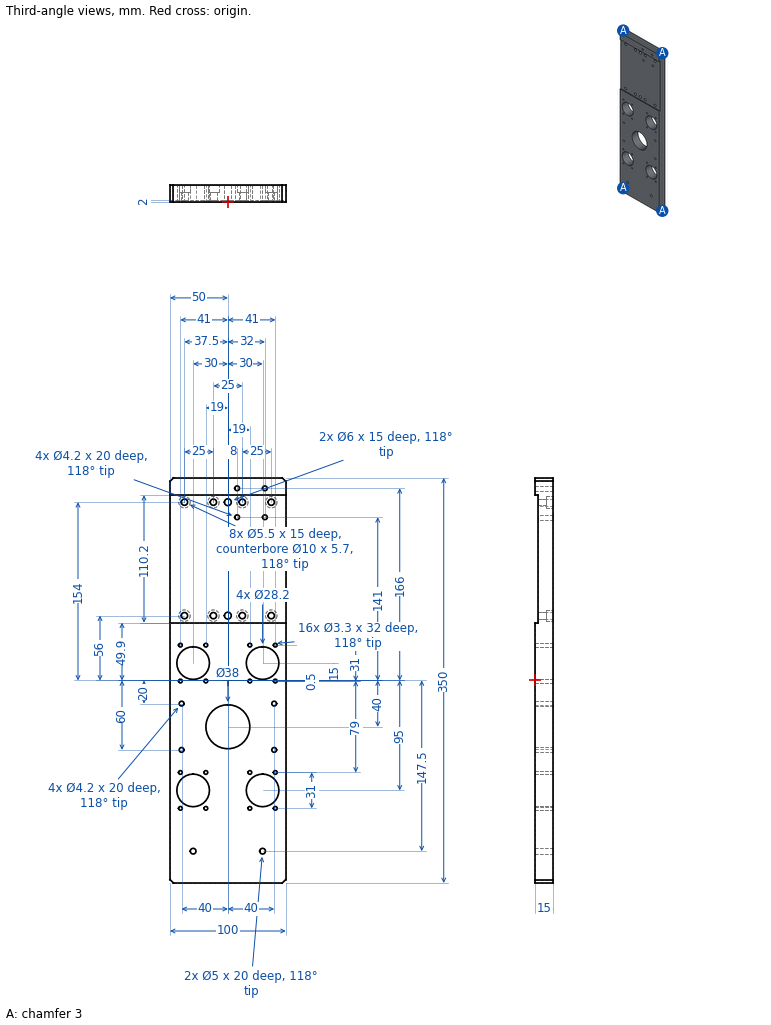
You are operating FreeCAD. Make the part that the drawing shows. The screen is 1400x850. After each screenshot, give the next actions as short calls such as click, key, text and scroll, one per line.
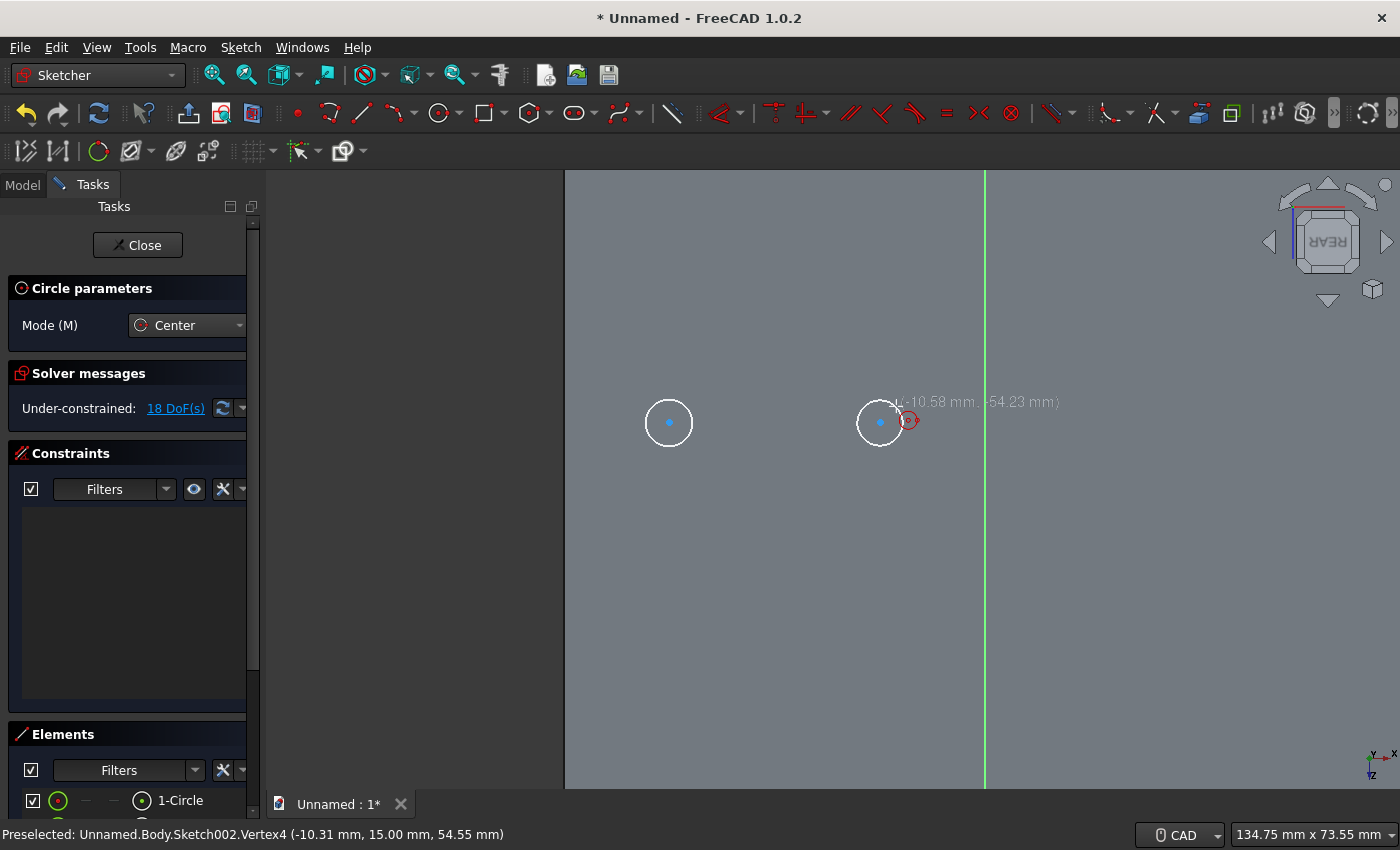
click(1090, 422)
click(1107, 406)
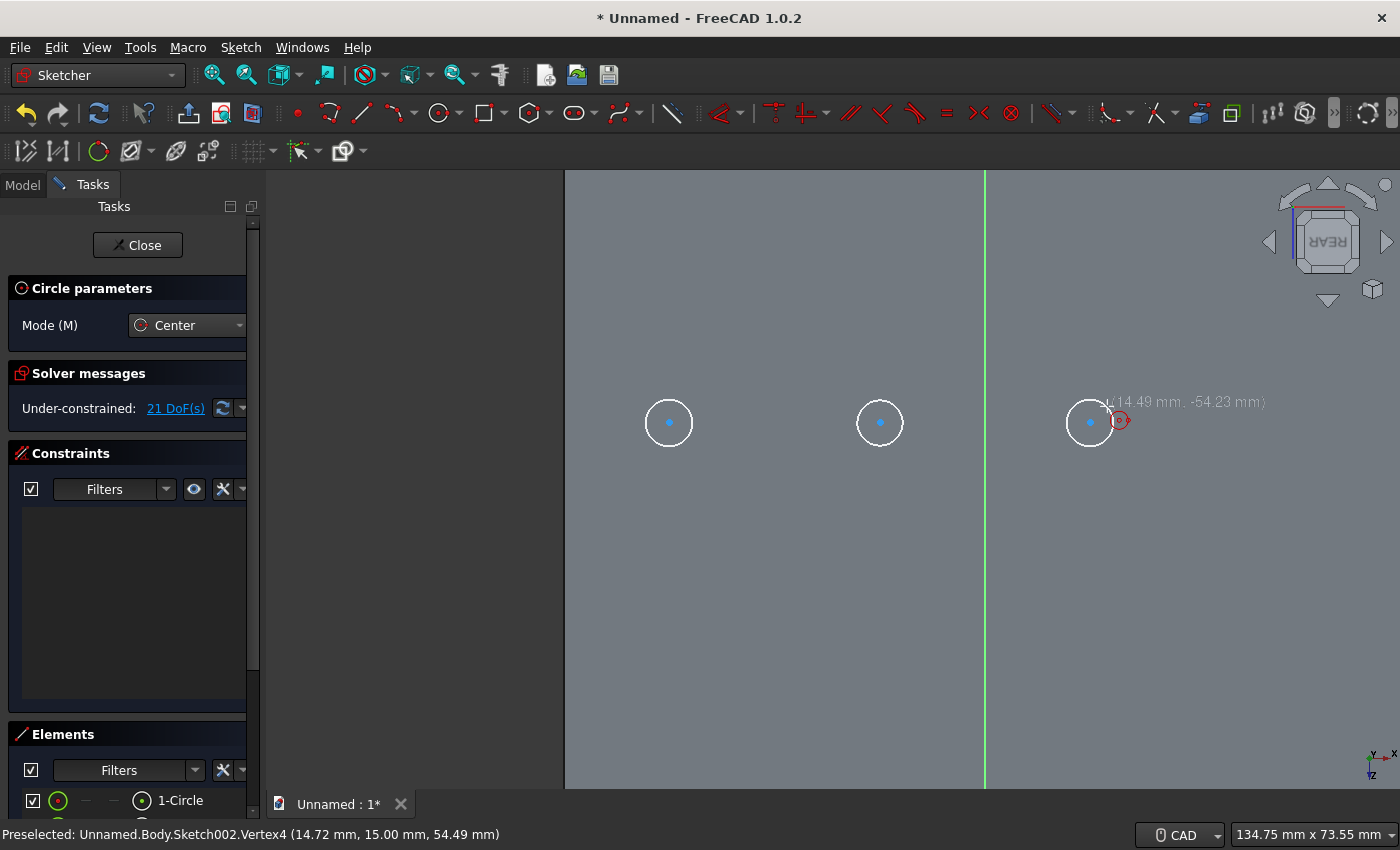
scroll(669, 423, down, 6)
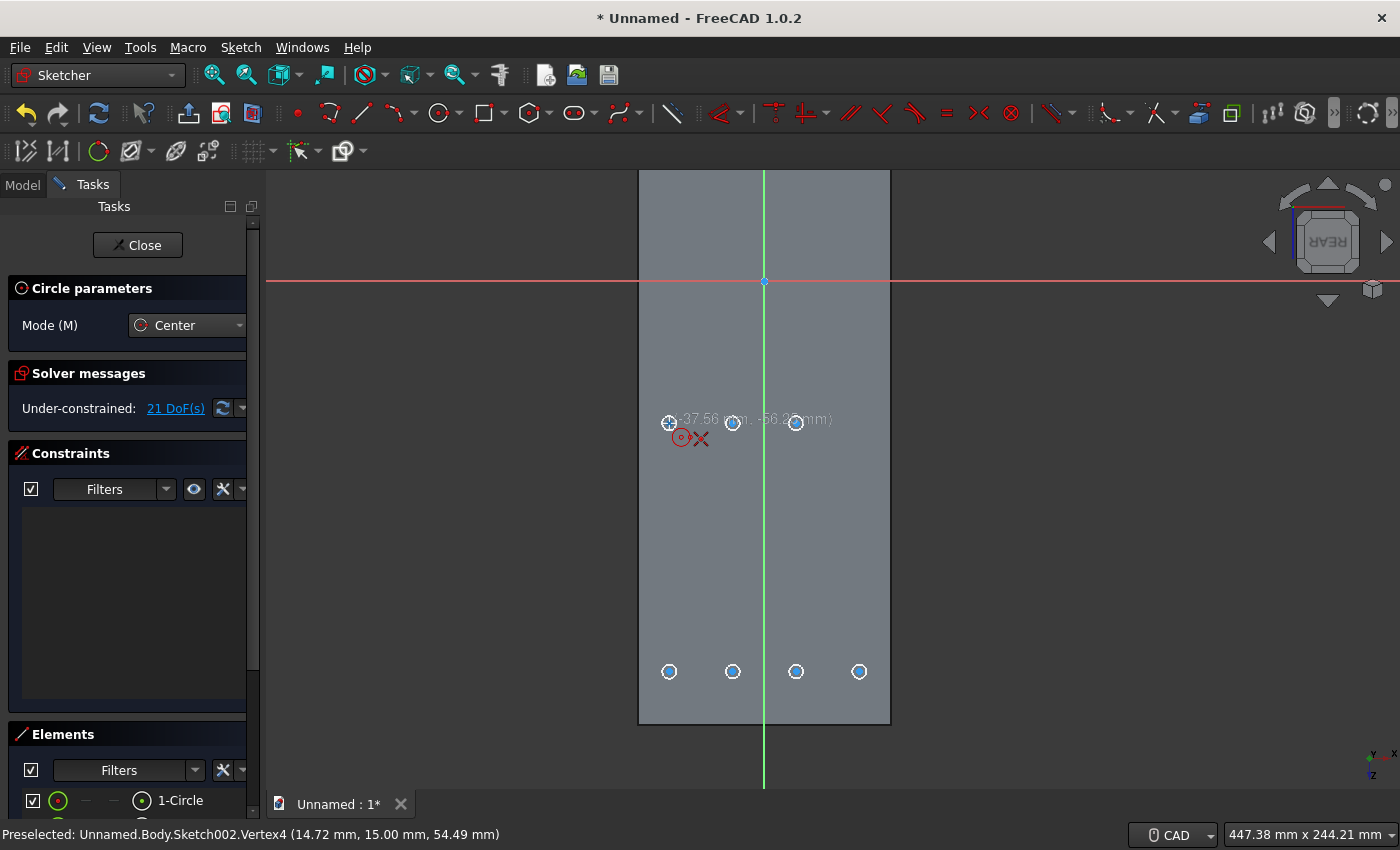
scroll(859, 423, up, 6)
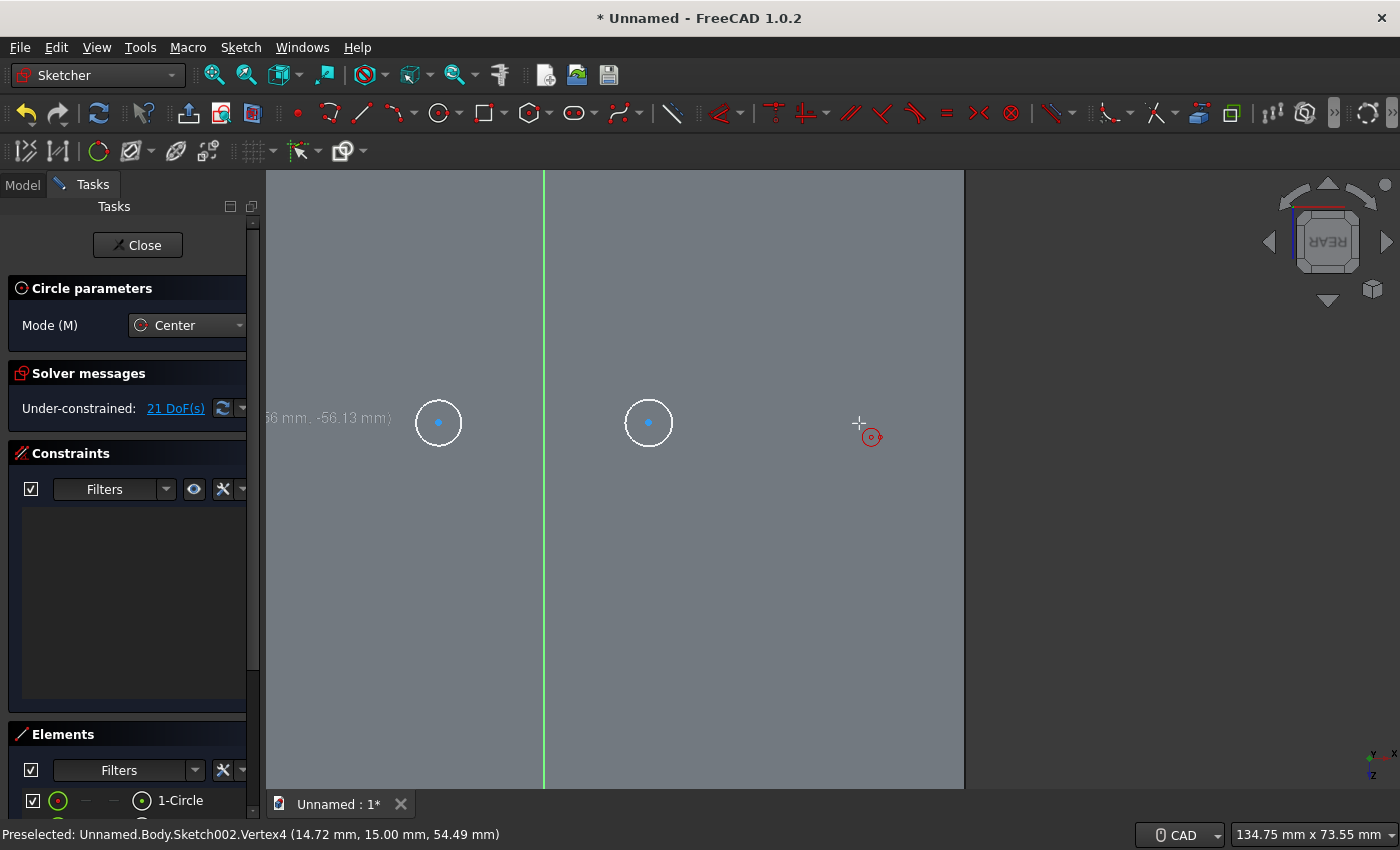
click(859, 422)
click(876, 406)
key(Escape)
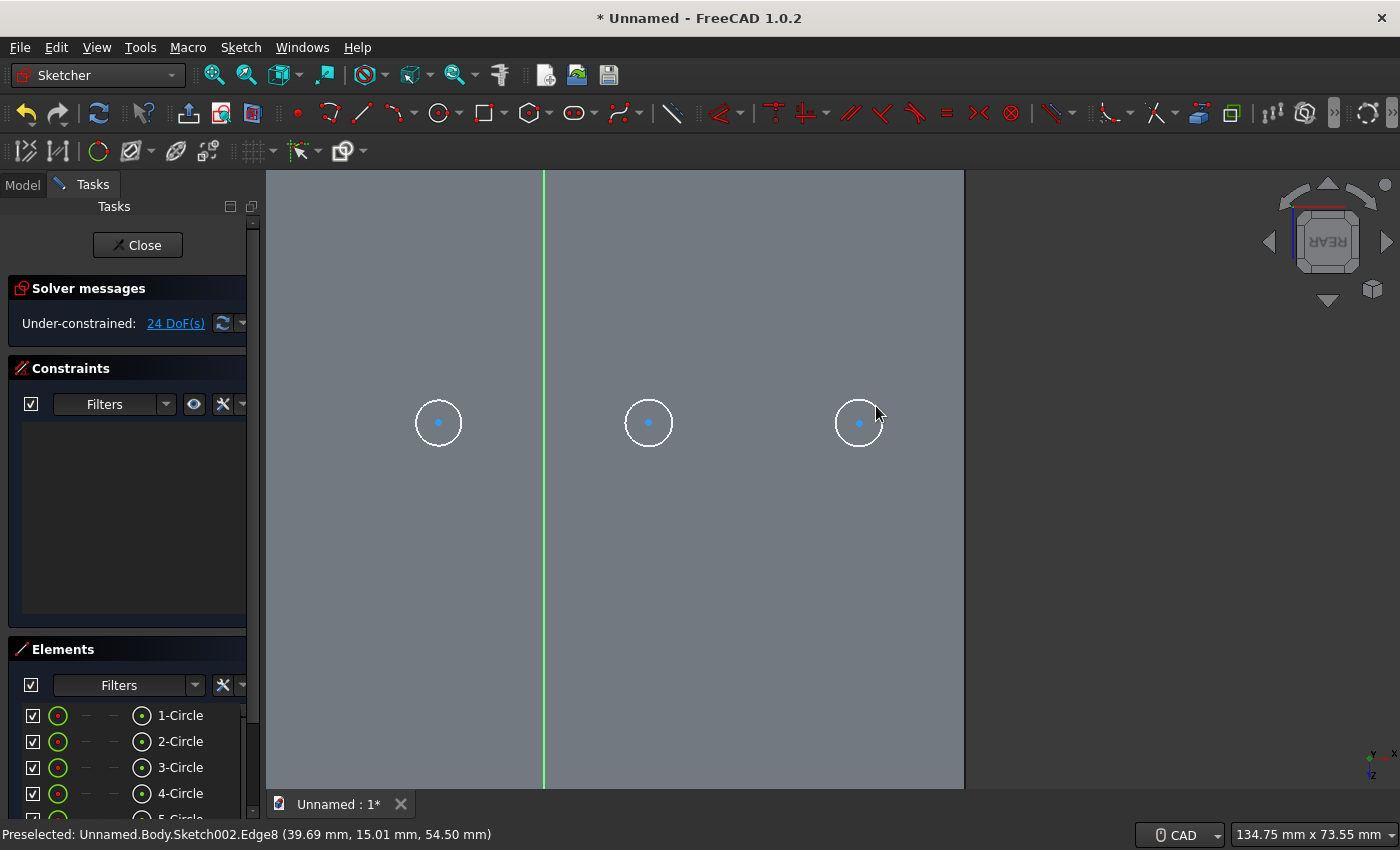
scroll(860, 423, down, 6)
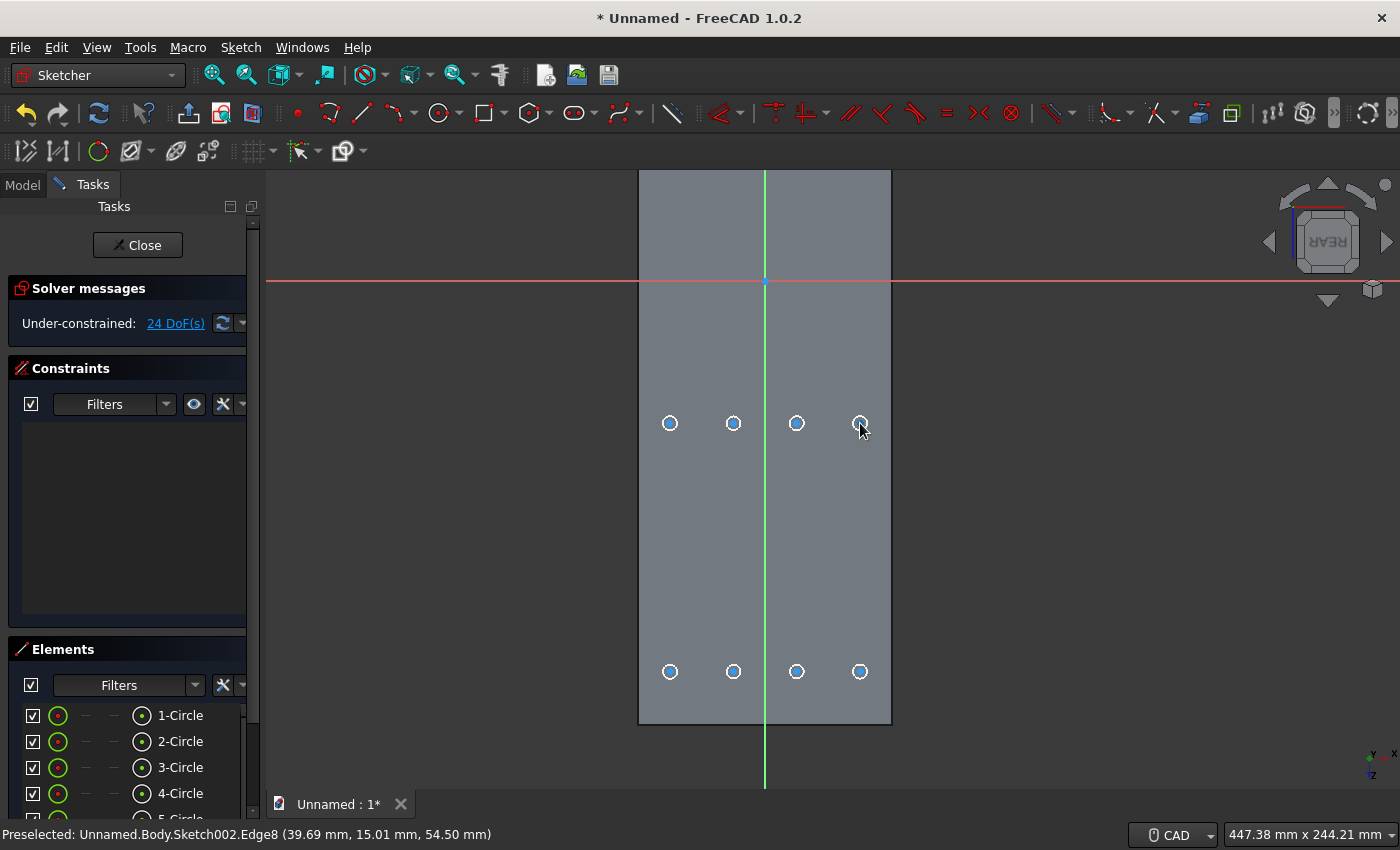
scroll(675, 667, up, 4)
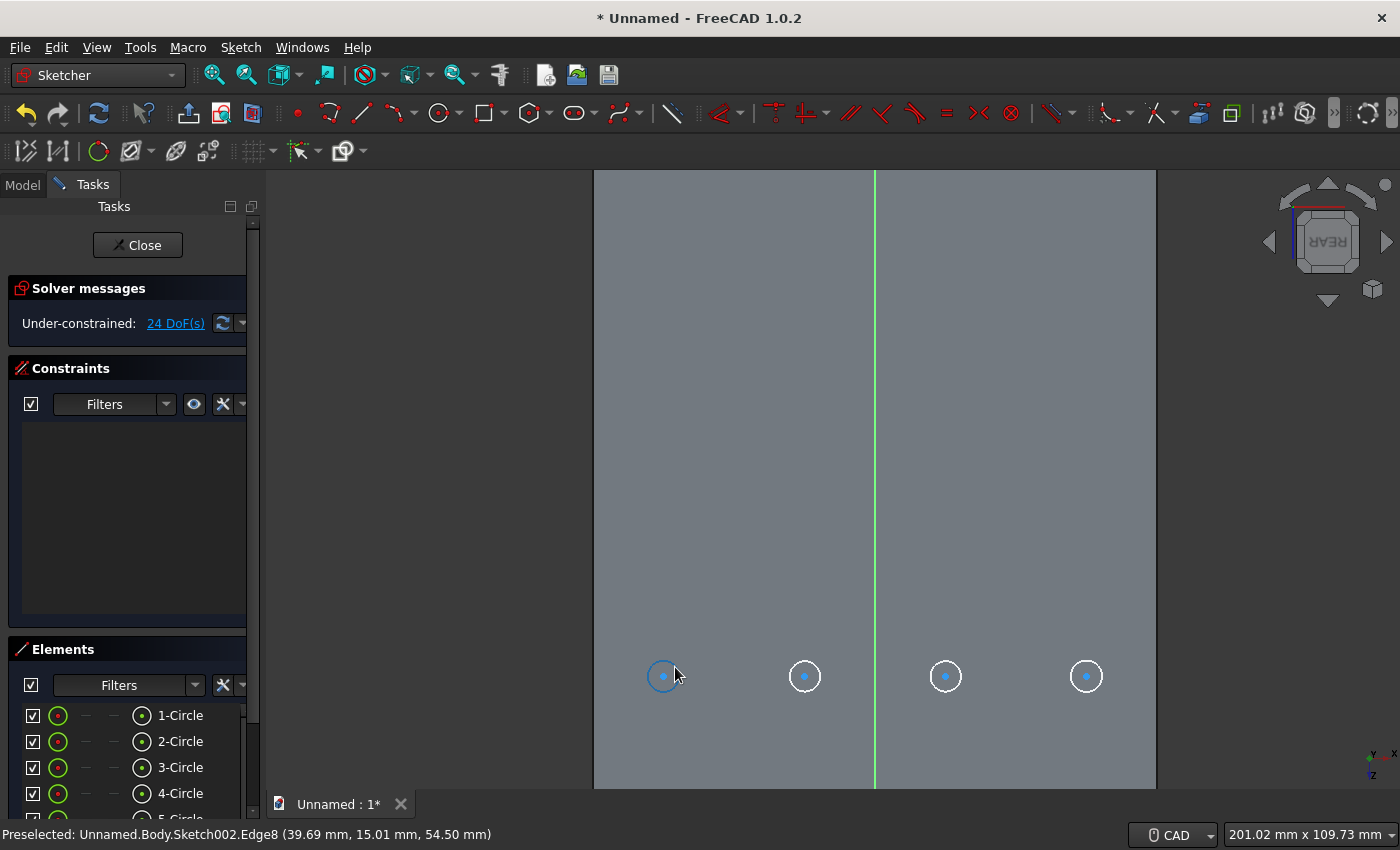
click(675, 665)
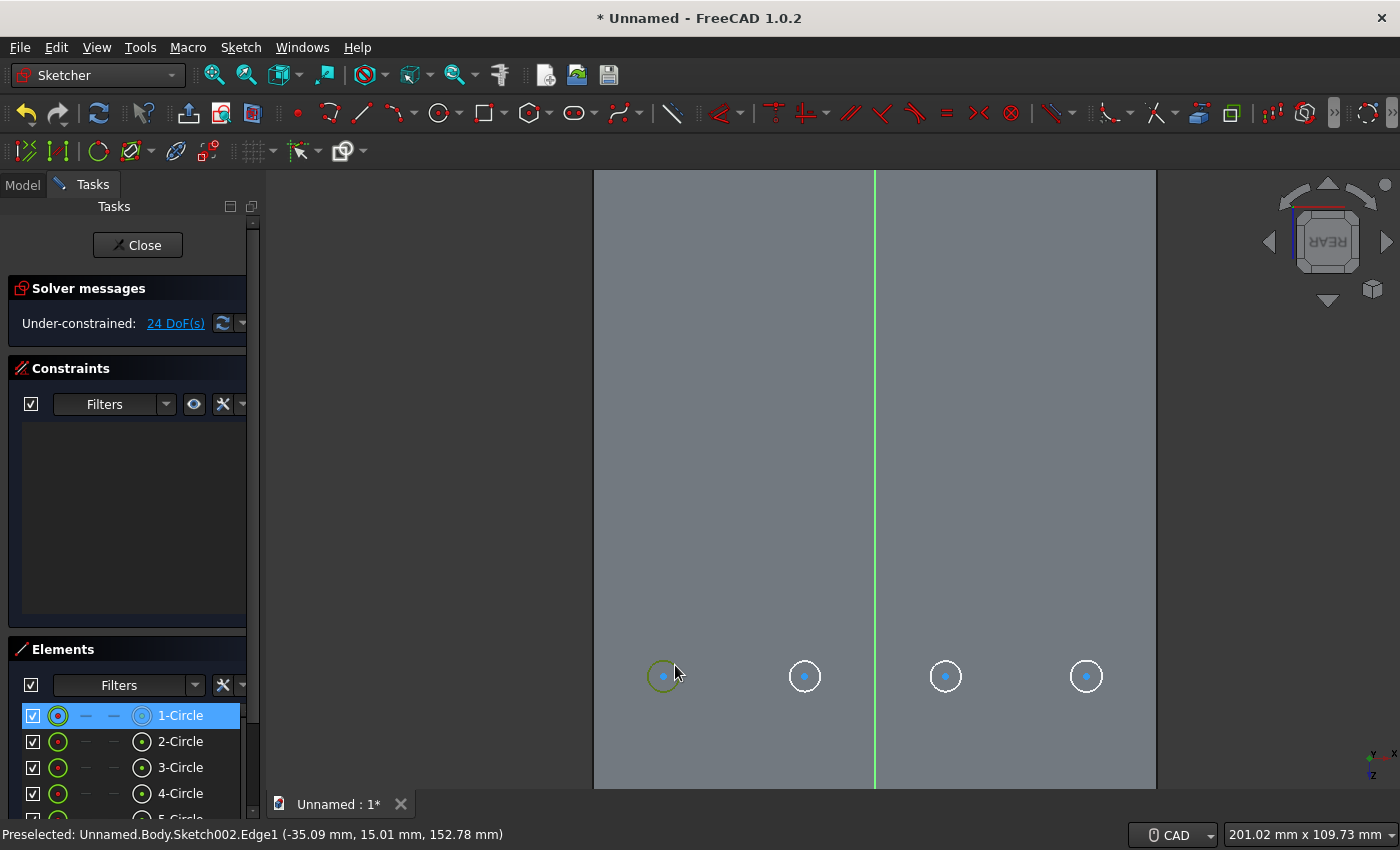
click(816, 666)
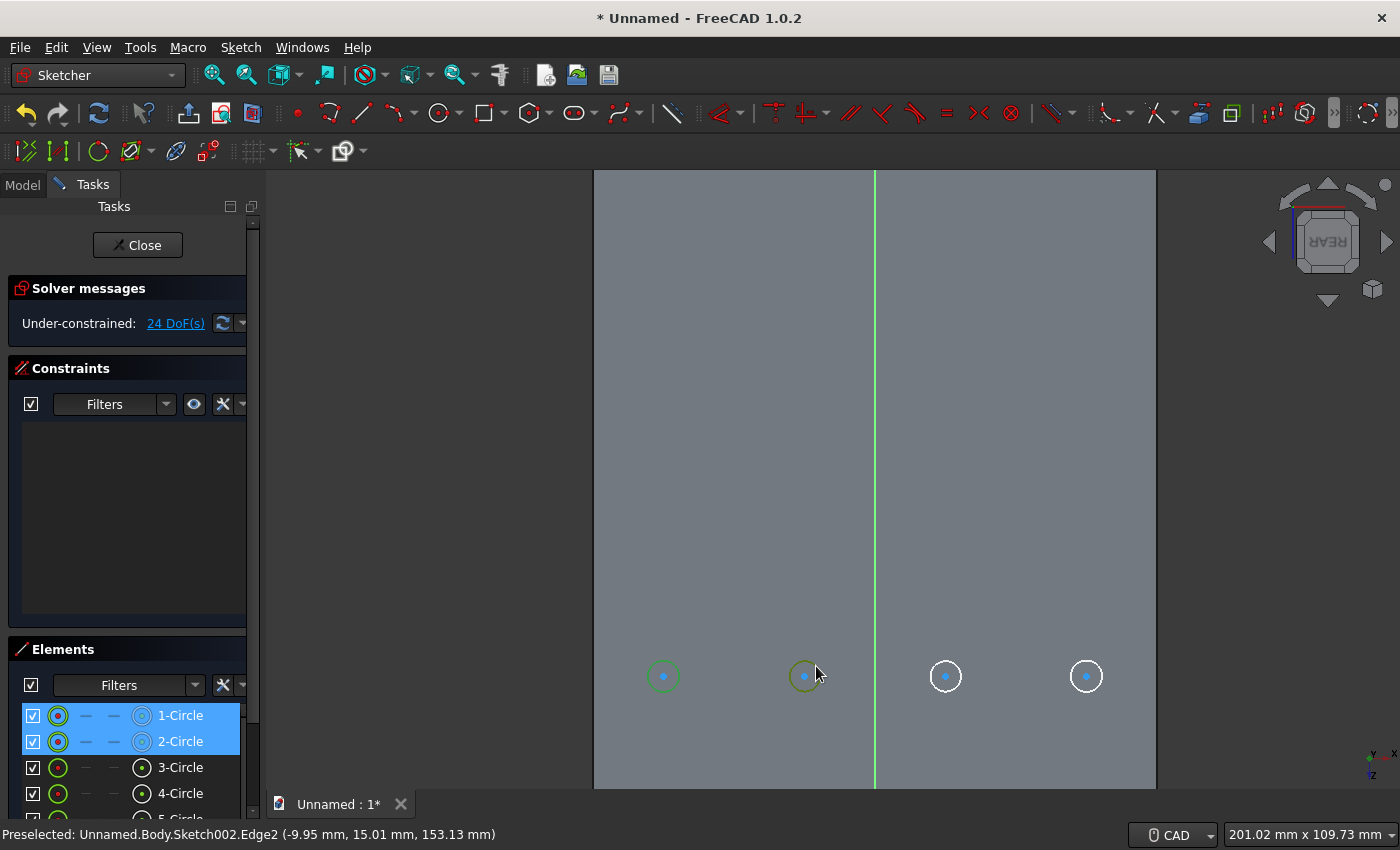
click(956, 666)